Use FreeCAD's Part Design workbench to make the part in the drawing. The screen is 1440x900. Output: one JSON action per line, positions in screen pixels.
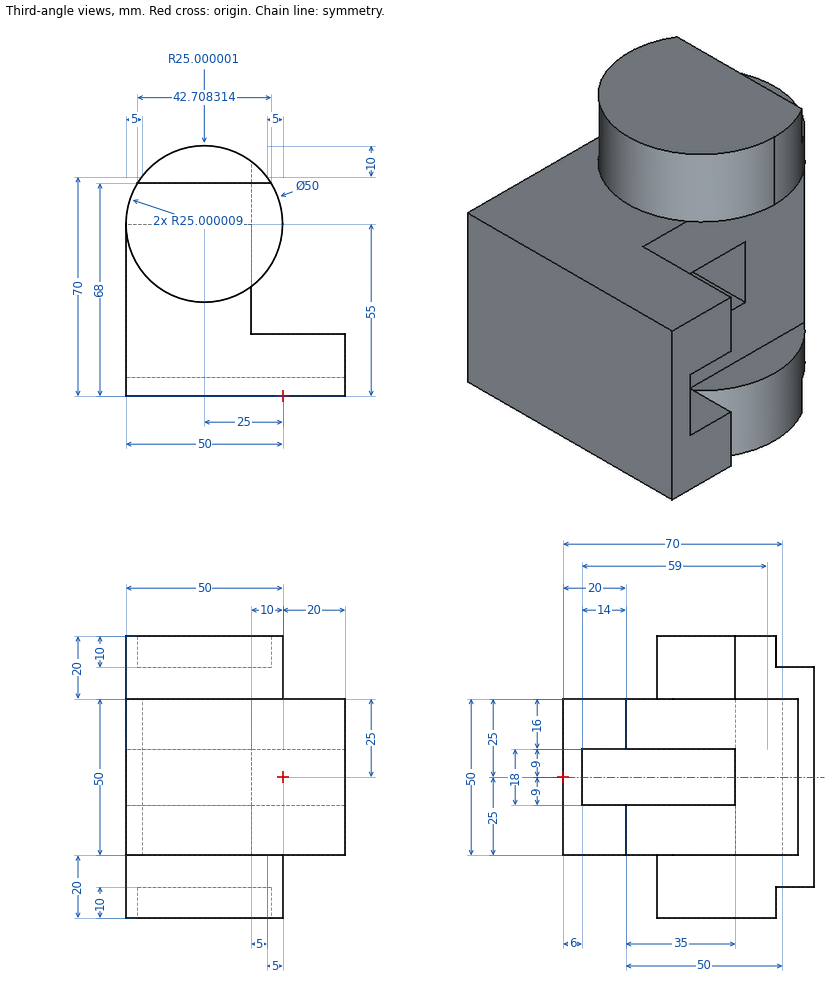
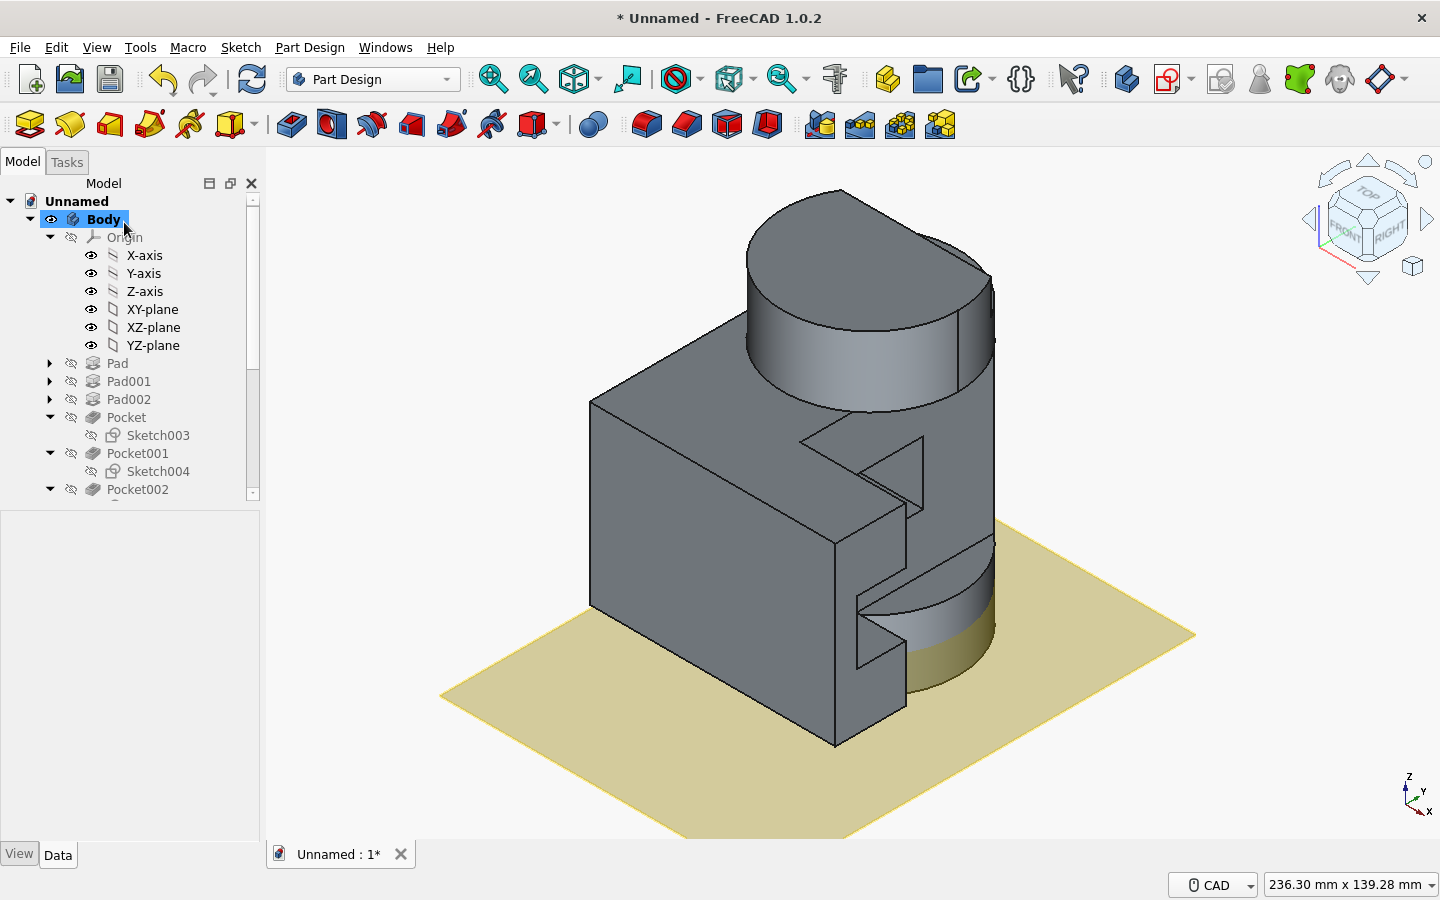
{"action": "scroll", "coordinate": [100, 341], "scroll_direction": "down", "scroll_amount": 3}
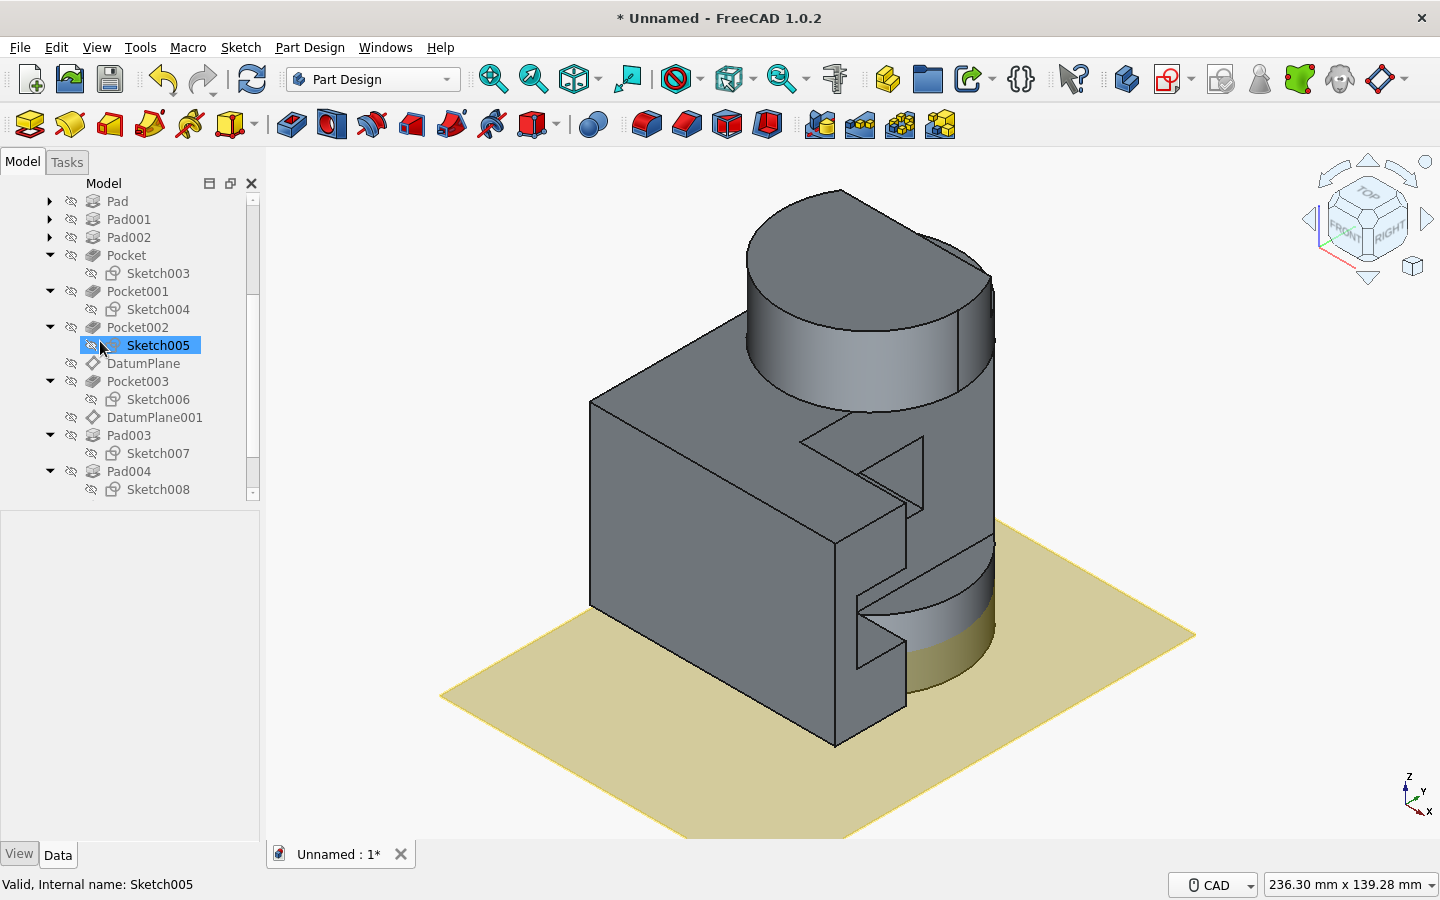
{"action": "scroll", "coordinate": [140, 341], "scroll_direction": "up", "scroll_amount": 15}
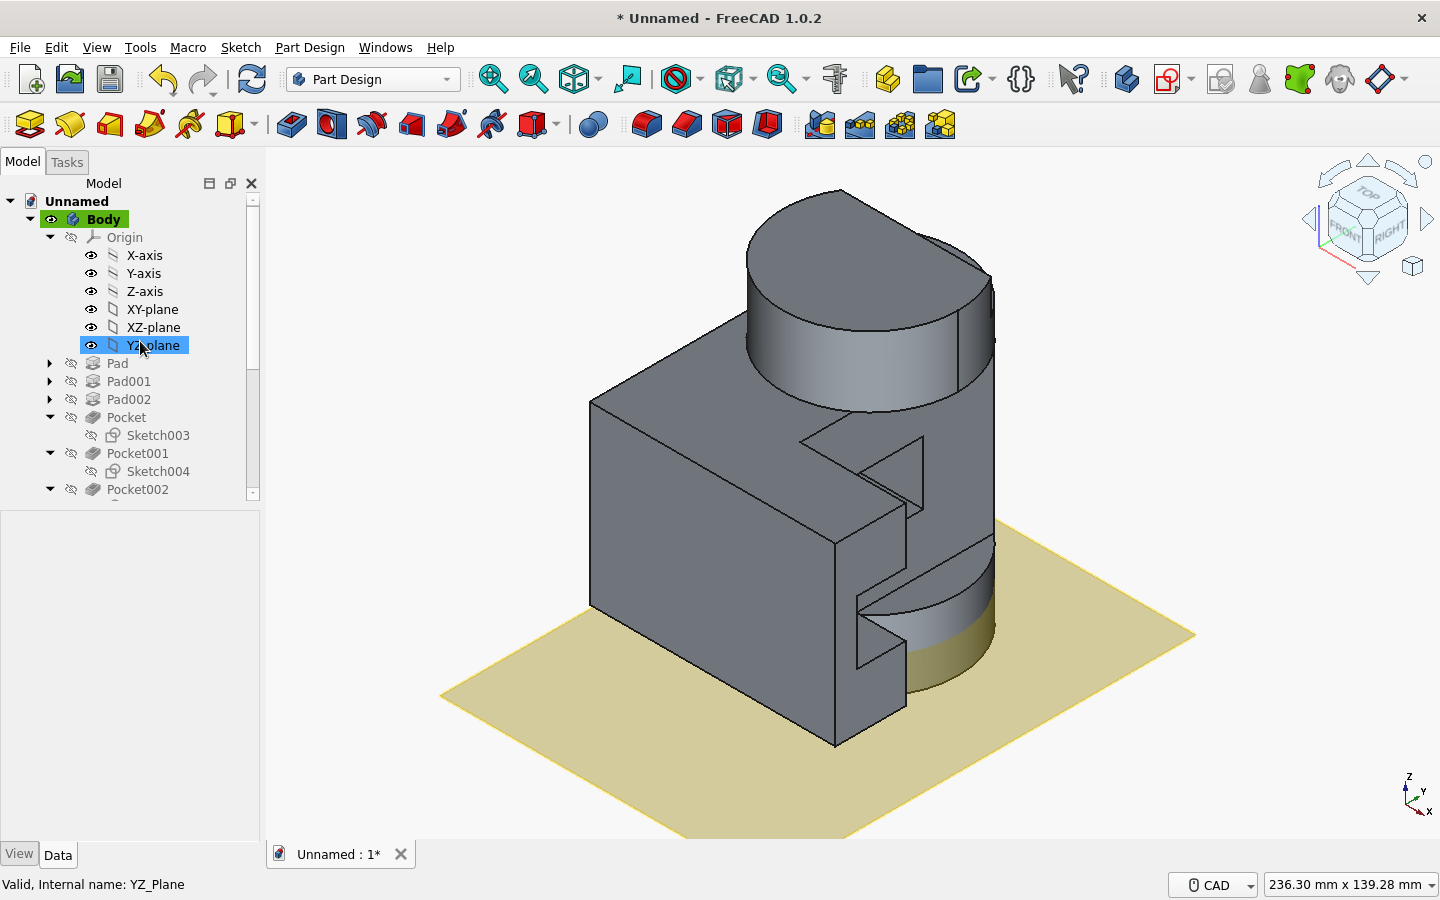
{"action": "scroll", "coordinate": [100, 341], "scroll_direction": "down", "scroll_amount": 6}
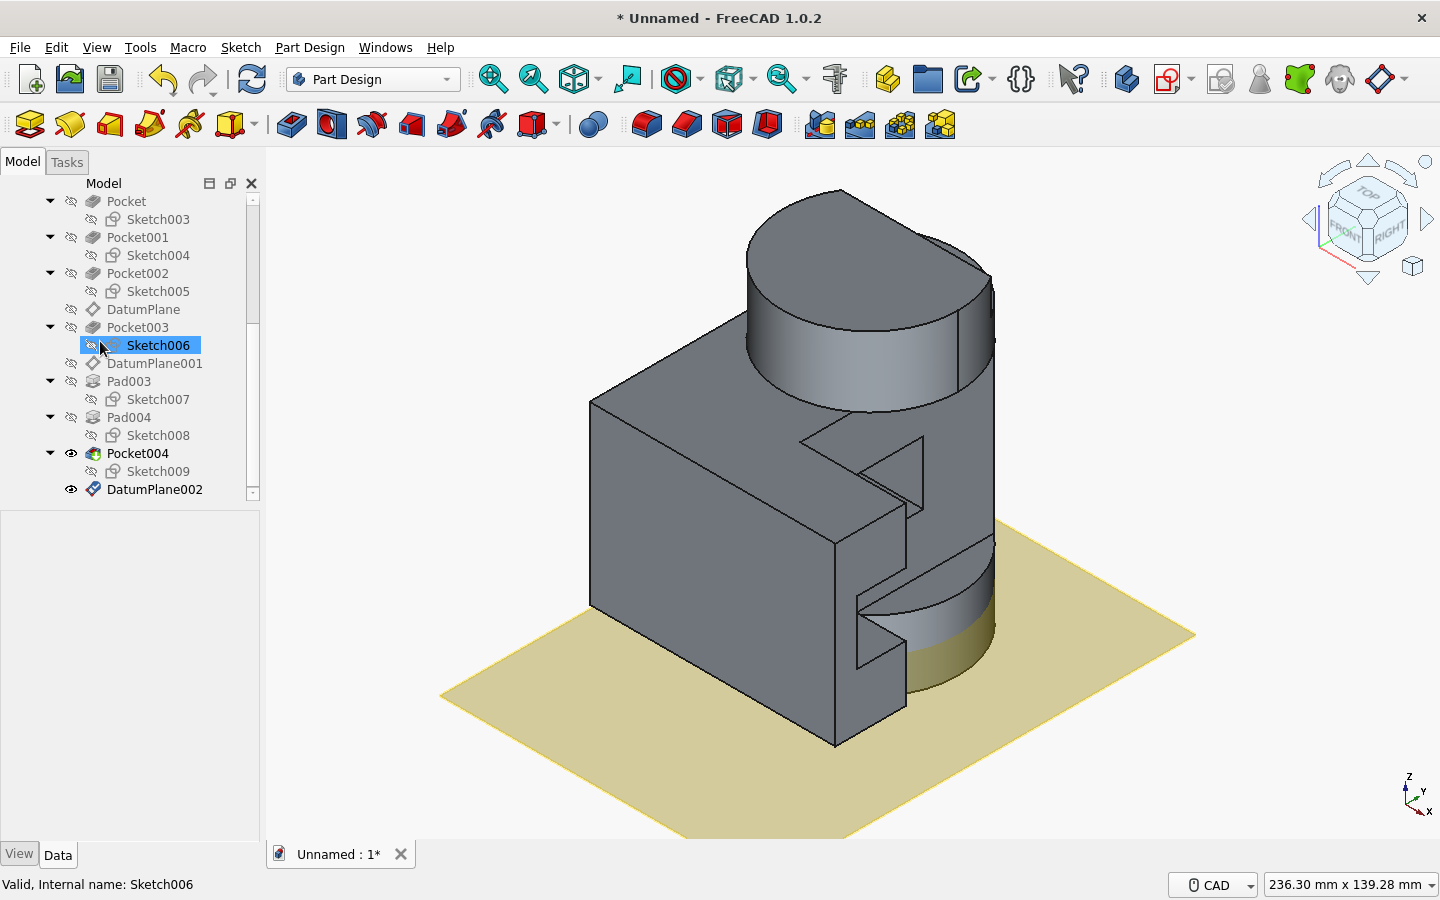
{"action": "left_click", "coordinate": [116, 489]}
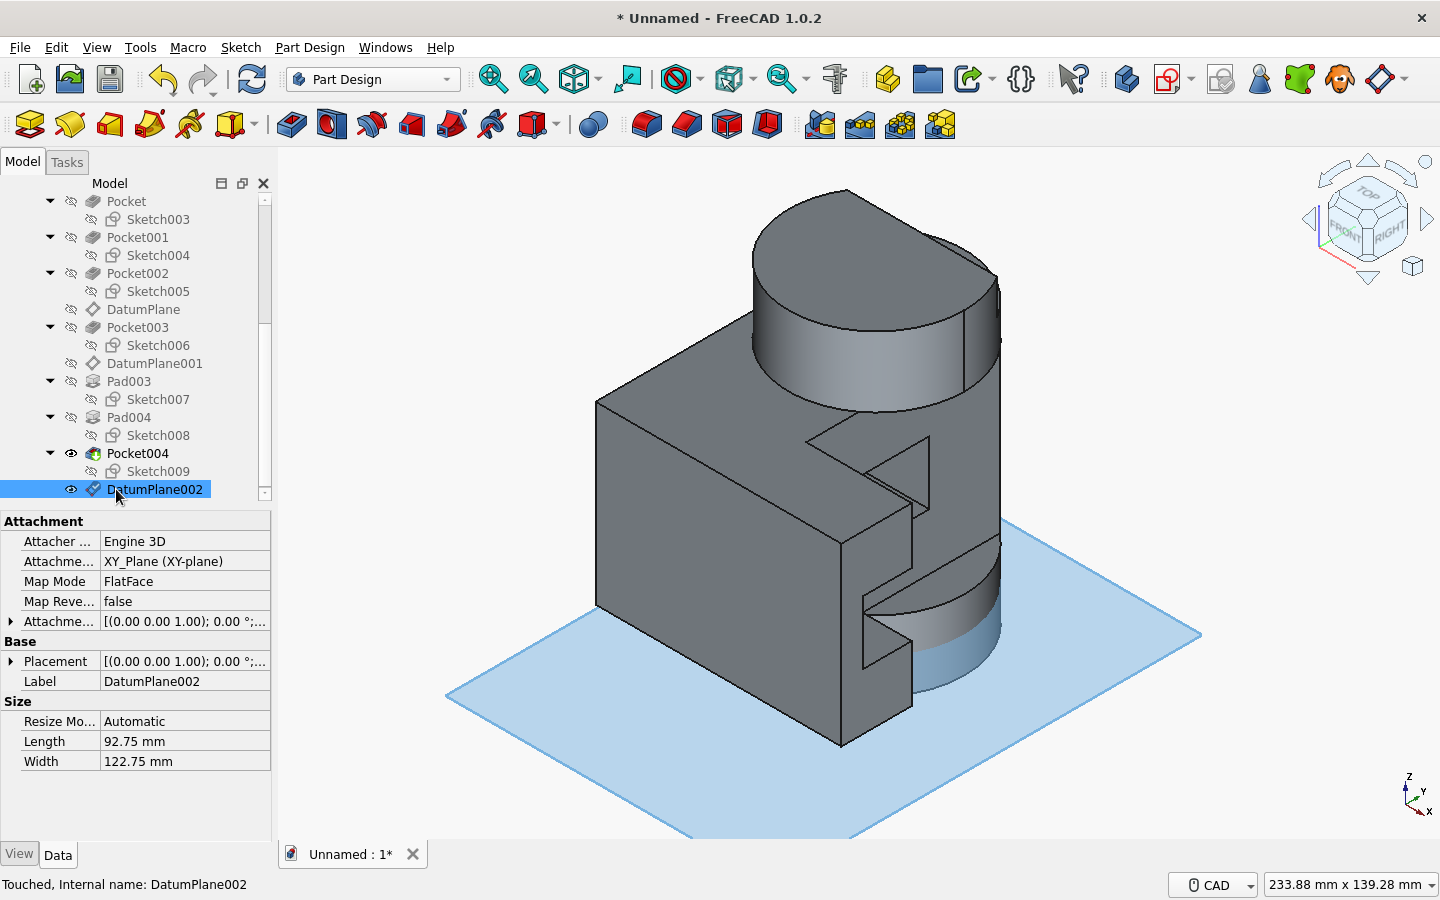
{"action": "left_click", "coordinate": [1168, 80]}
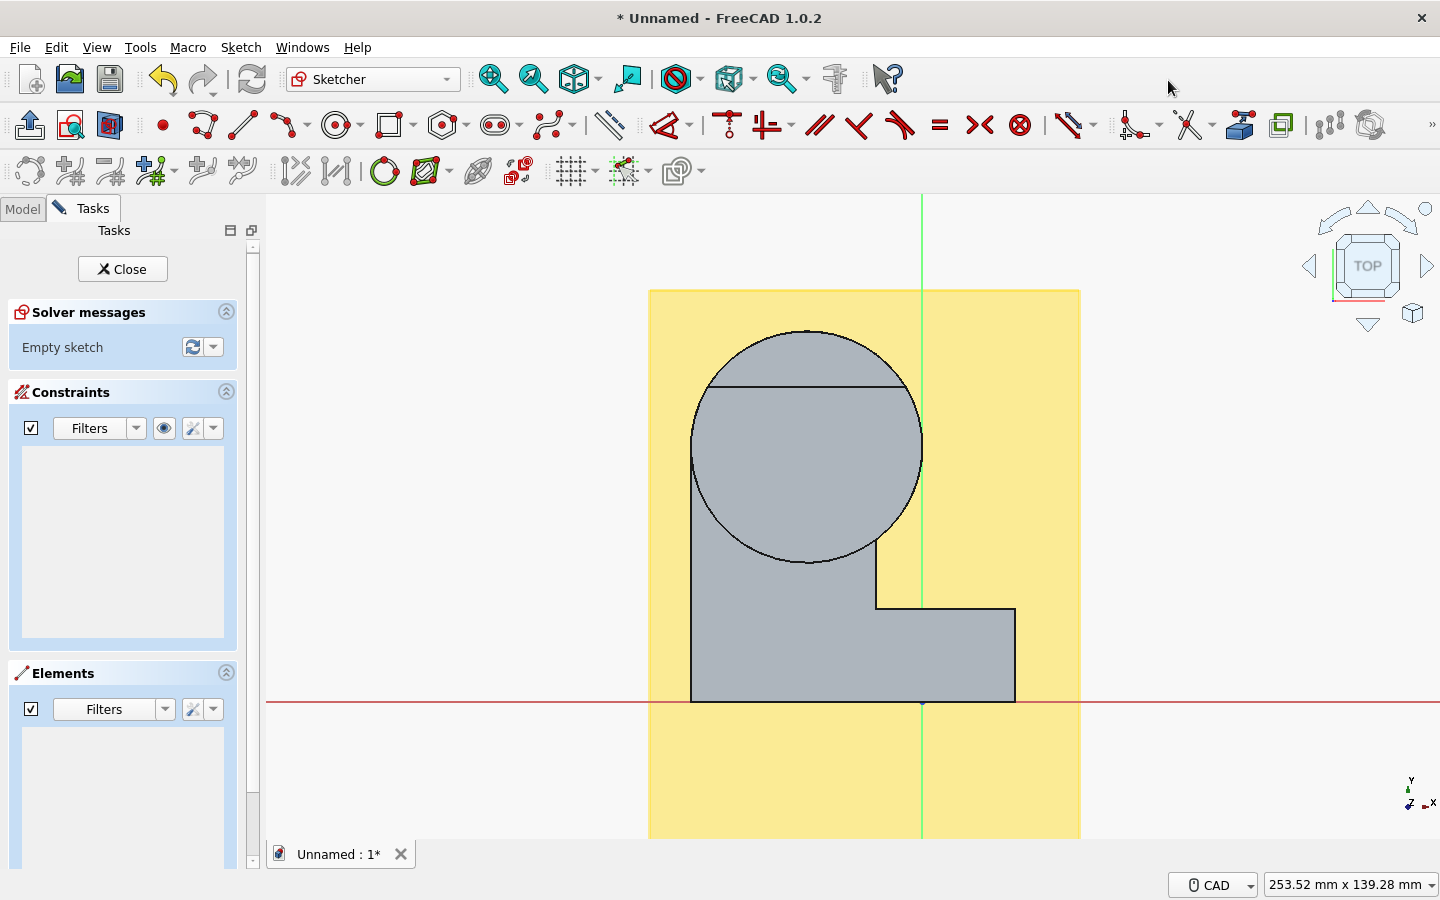
{"action": "key", "text": "q s"}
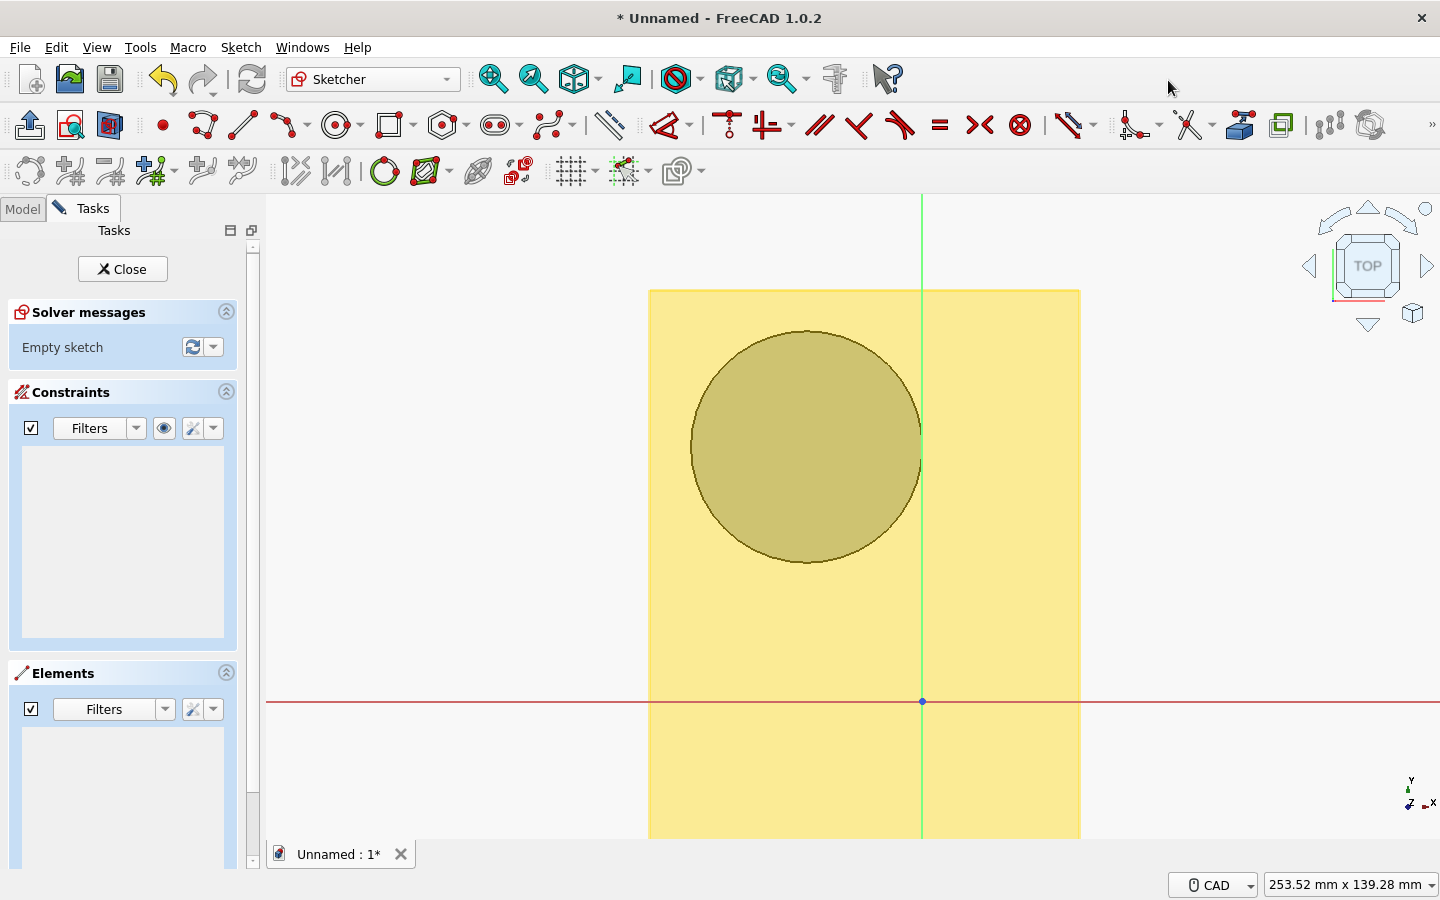
{"action": "key", "text": "g l"}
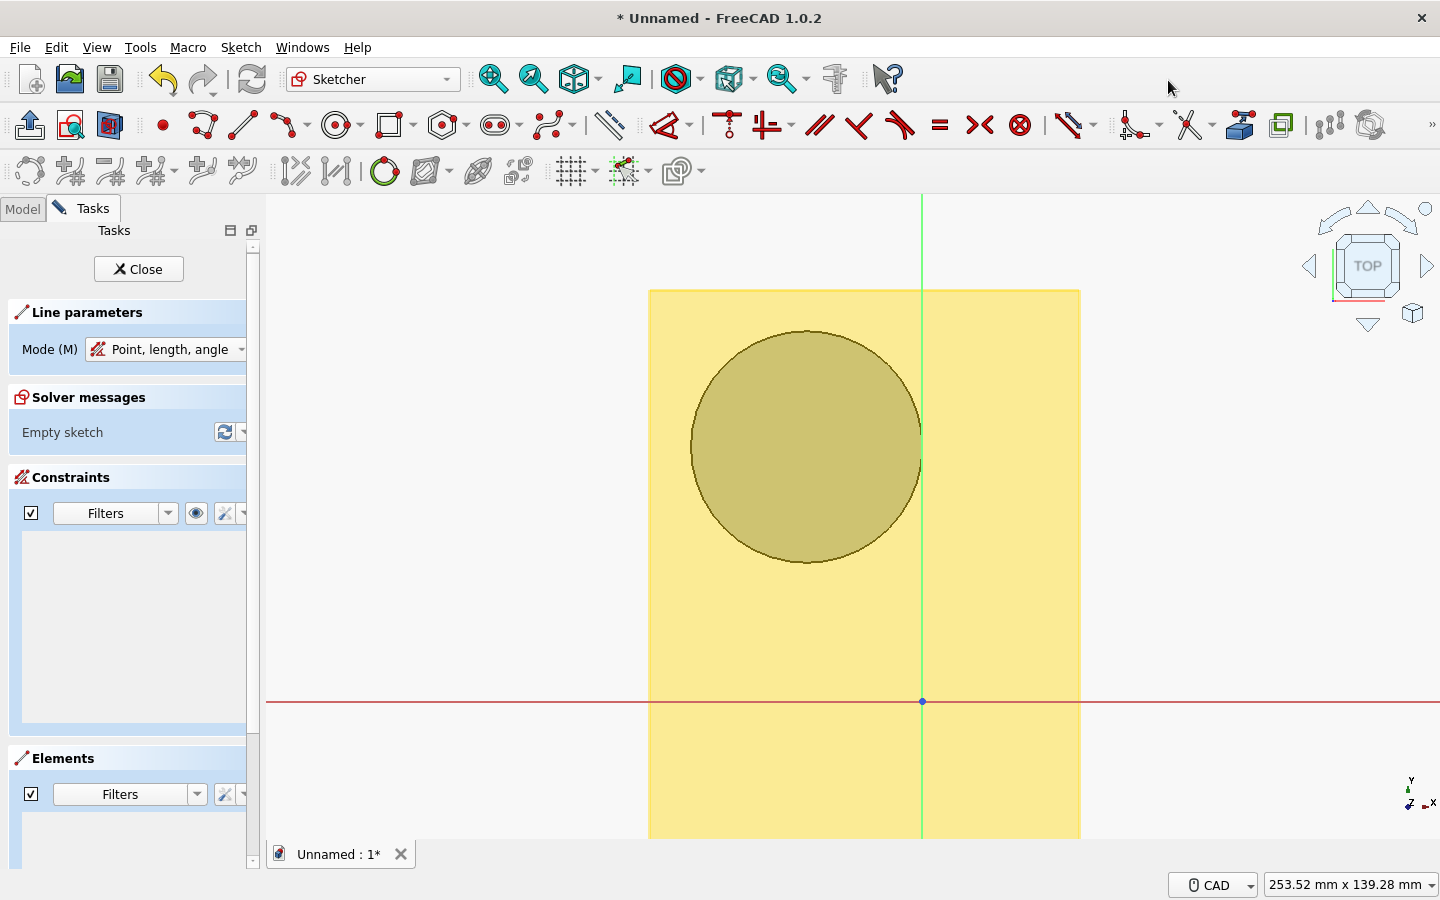
{"action": "left_click", "coordinate": [906, 387]}
{"action": "left_click", "coordinate": [708, 387]}